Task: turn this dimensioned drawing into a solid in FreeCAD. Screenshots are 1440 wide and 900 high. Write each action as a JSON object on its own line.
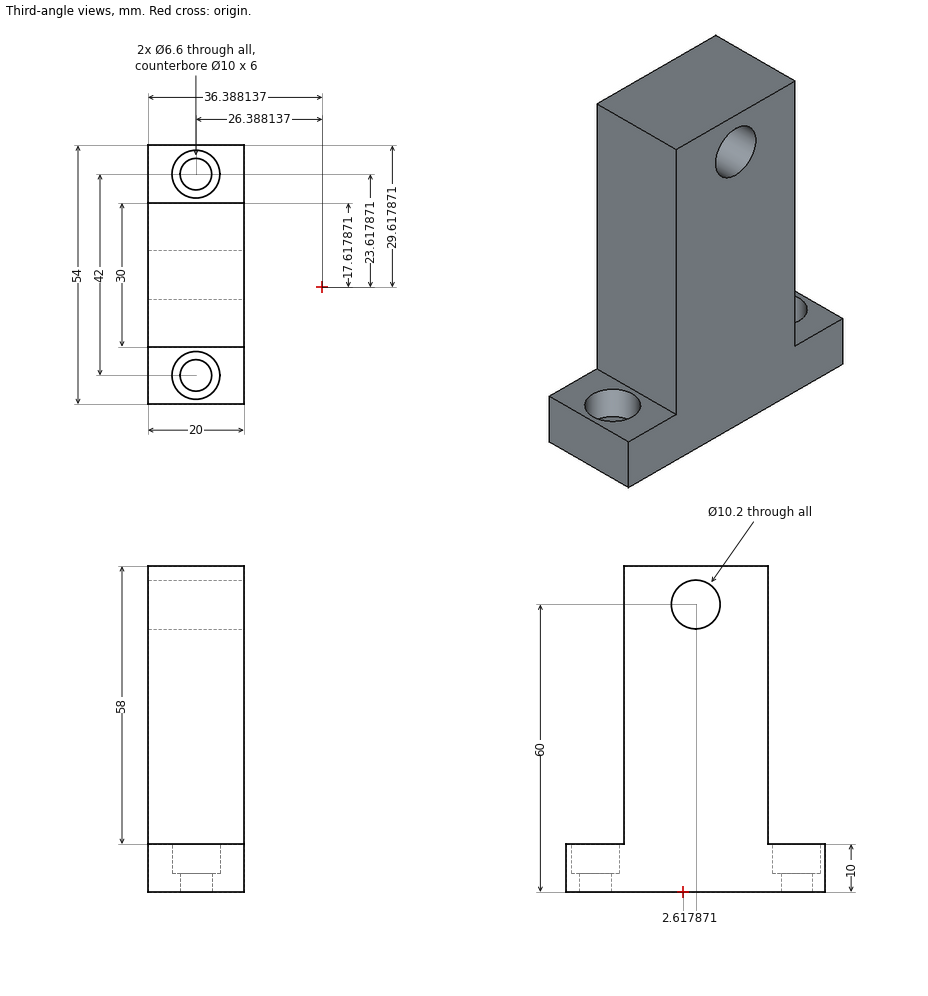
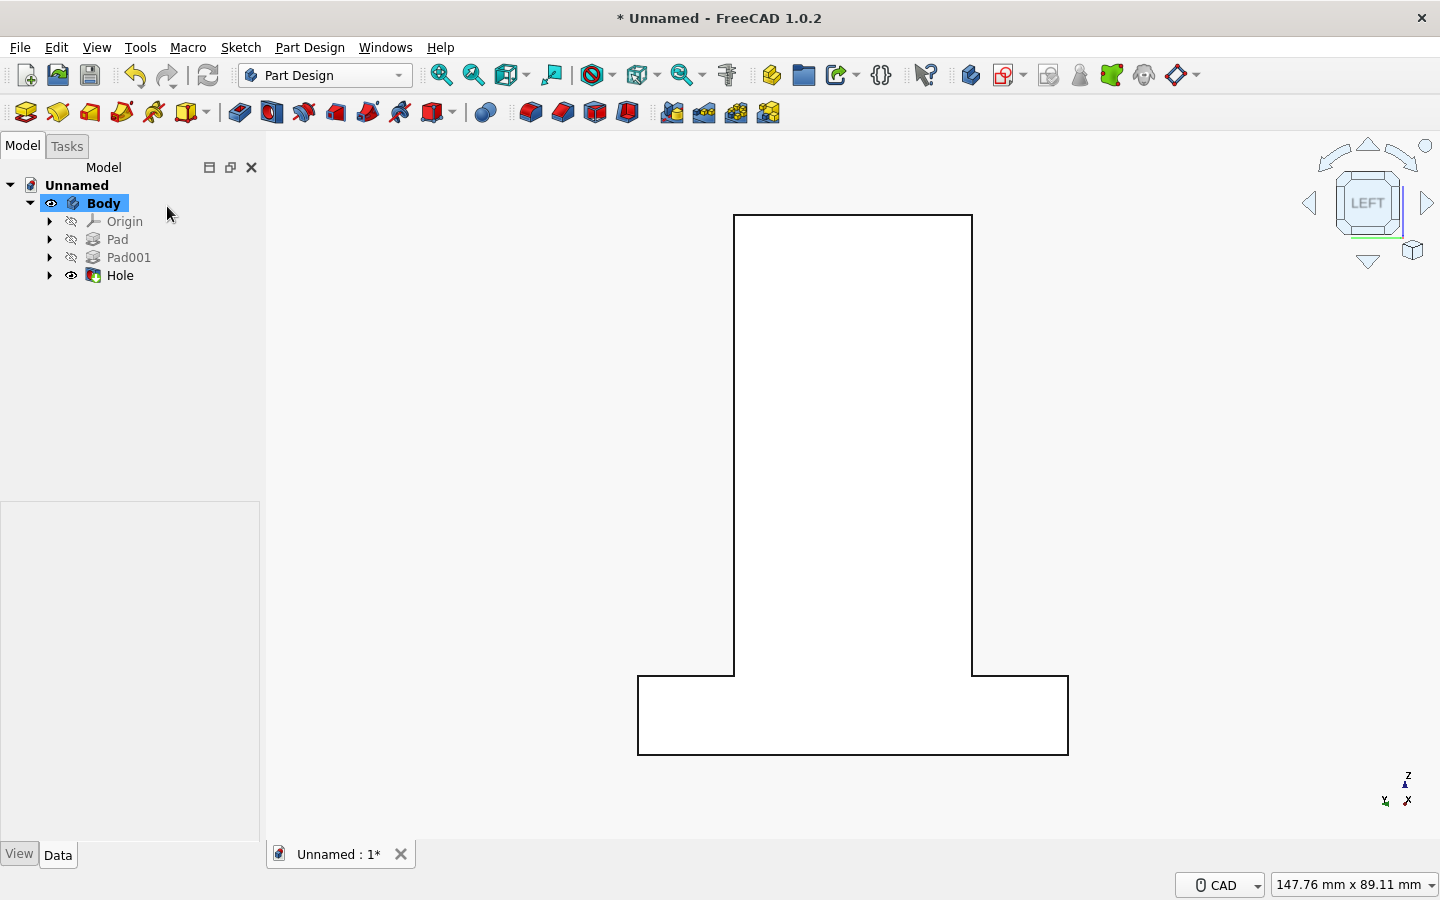
{"action": "left_click", "coordinate": [853, 407]}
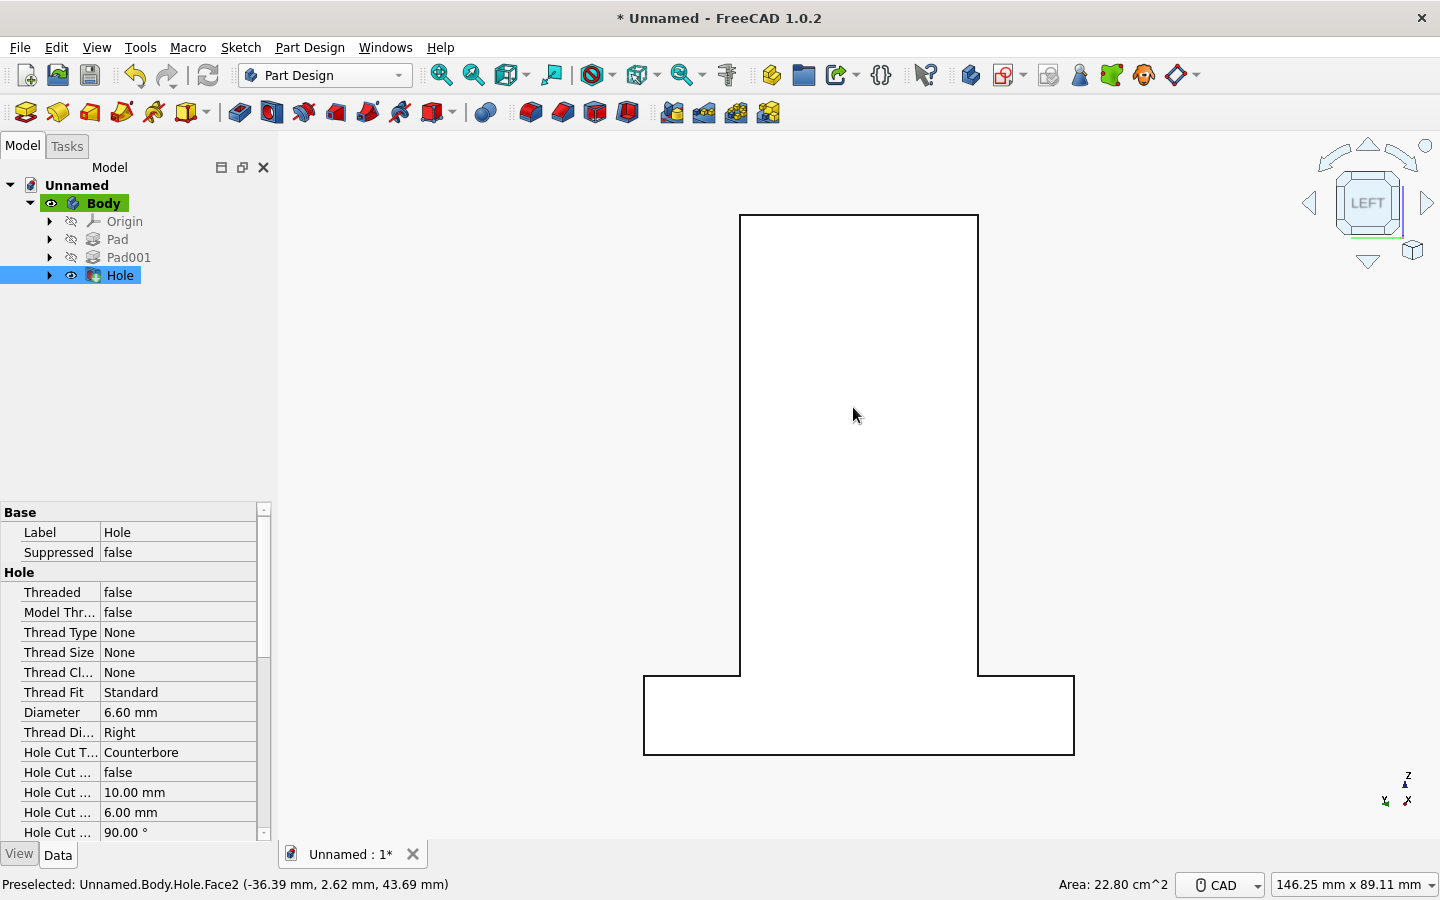
{"action": "left_click", "coordinate": [1004, 76]}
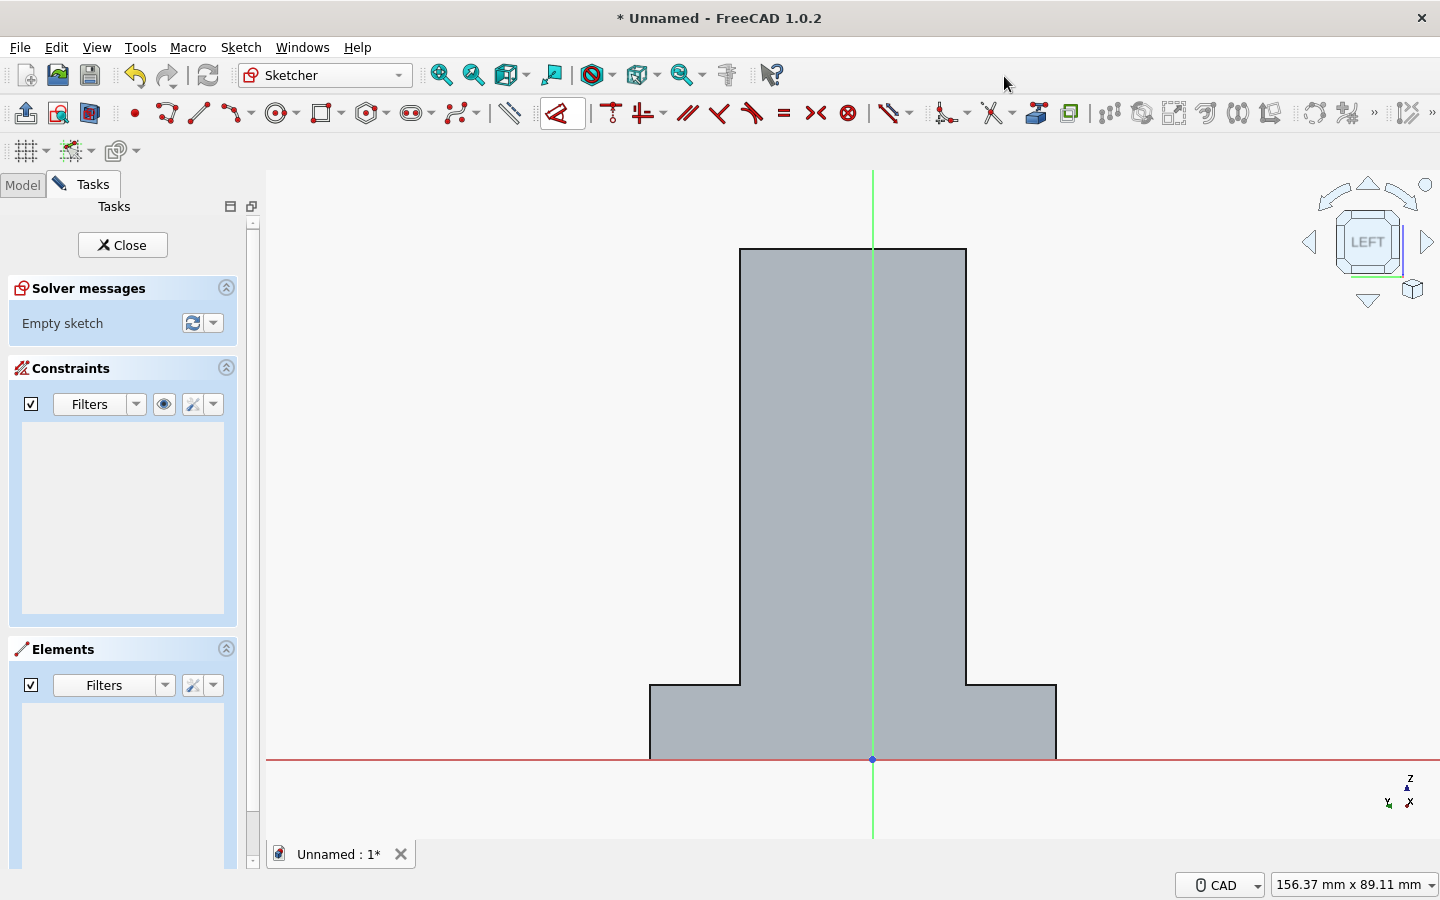
{"action": "scroll", "coordinate": [867, 271], "scroll_direction": "up", "scroll_amount": 9}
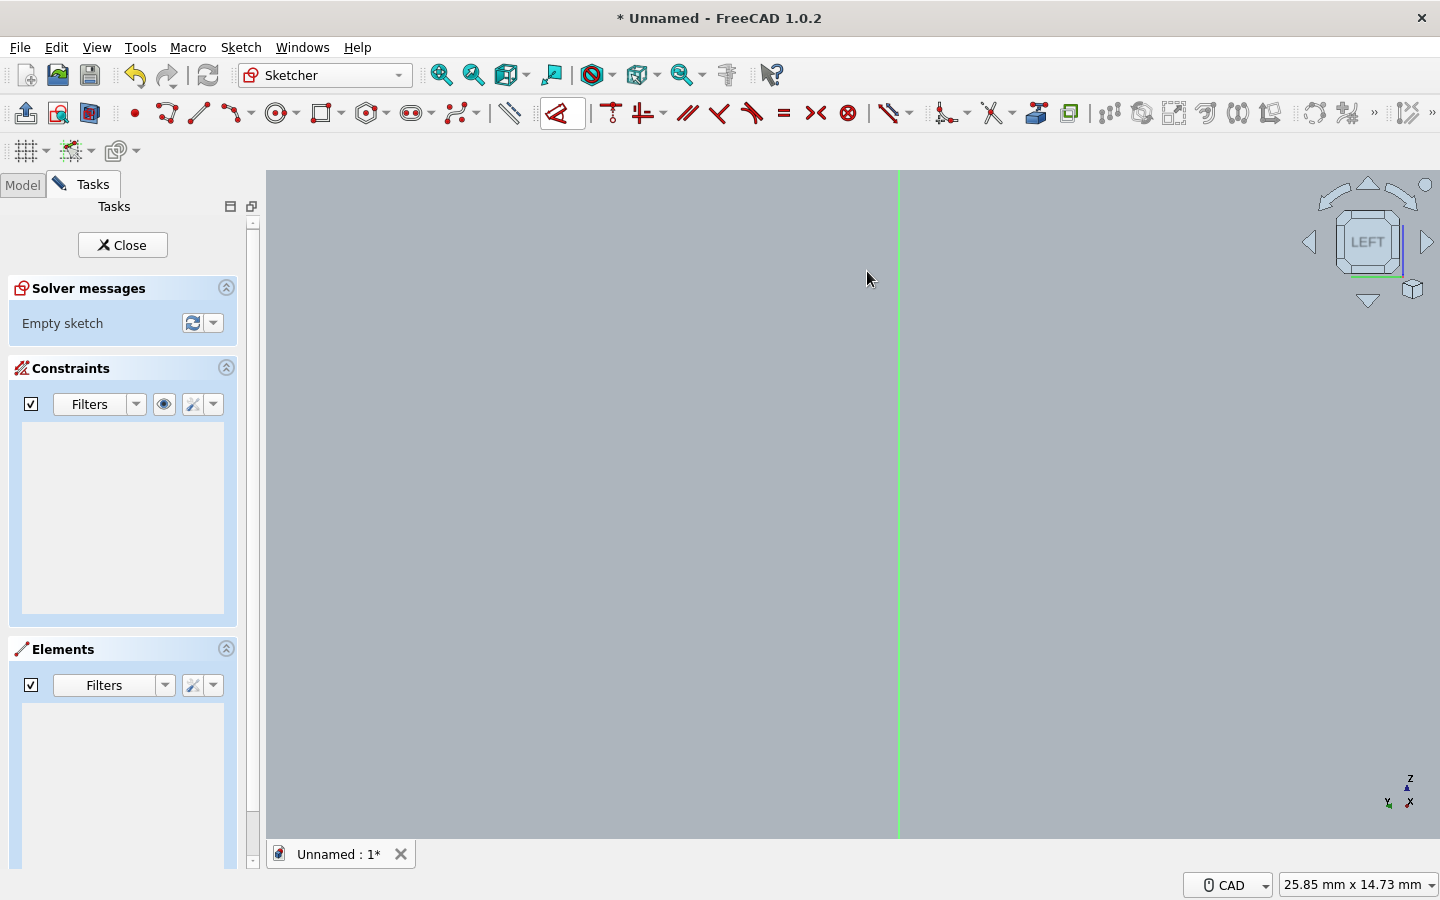
{"action": "left_click", "coordinate": [276, 114]}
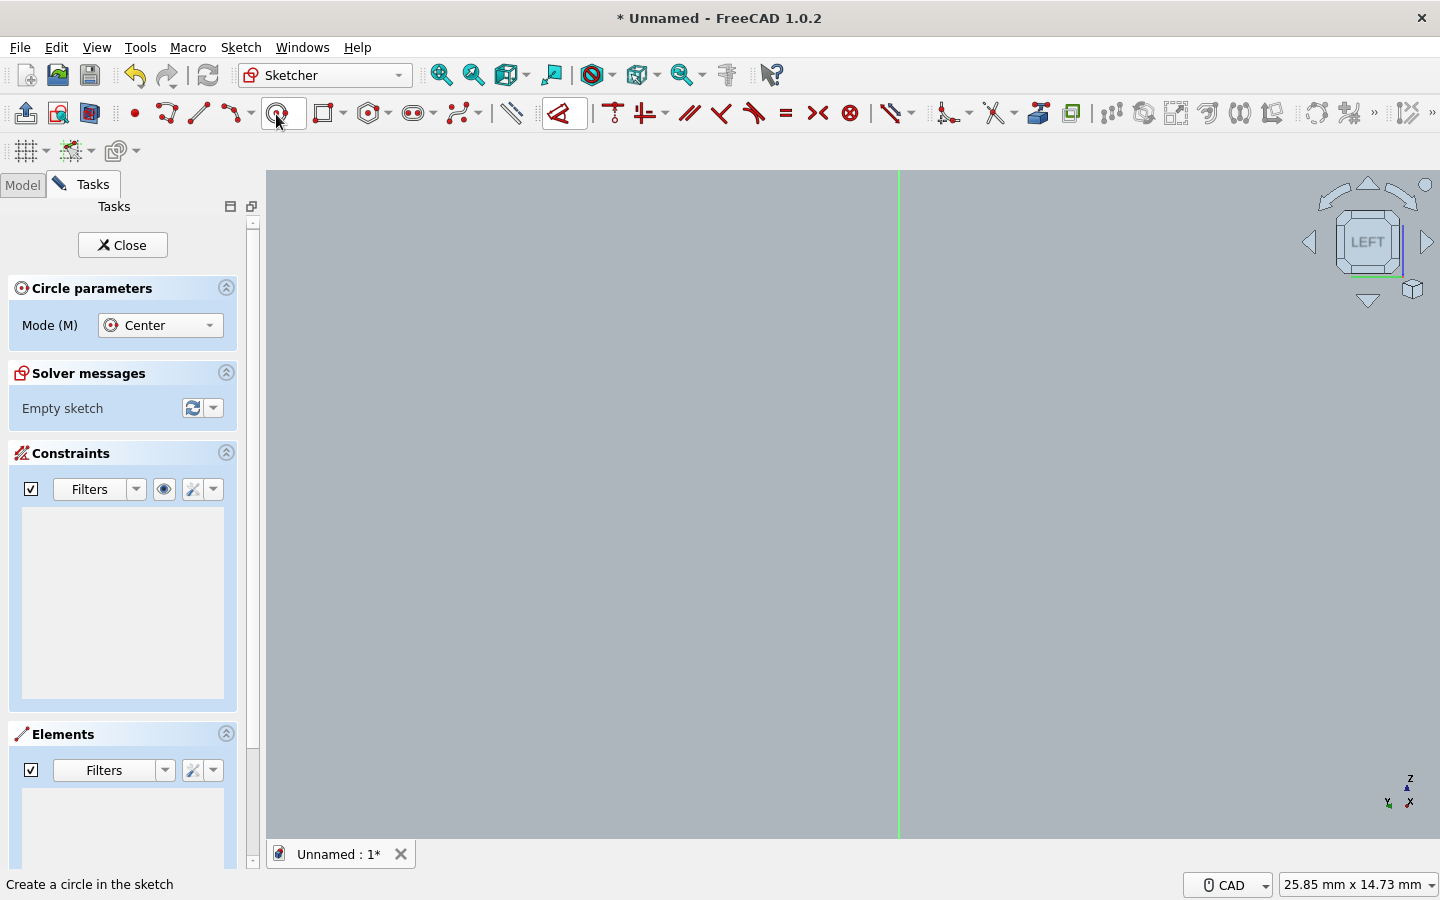
{"action": "left_click", "coordinate": [780, 502]}
{"action": "left_click", "coordinate": [944, 338]}
{"action": "key", "text": "Escape"}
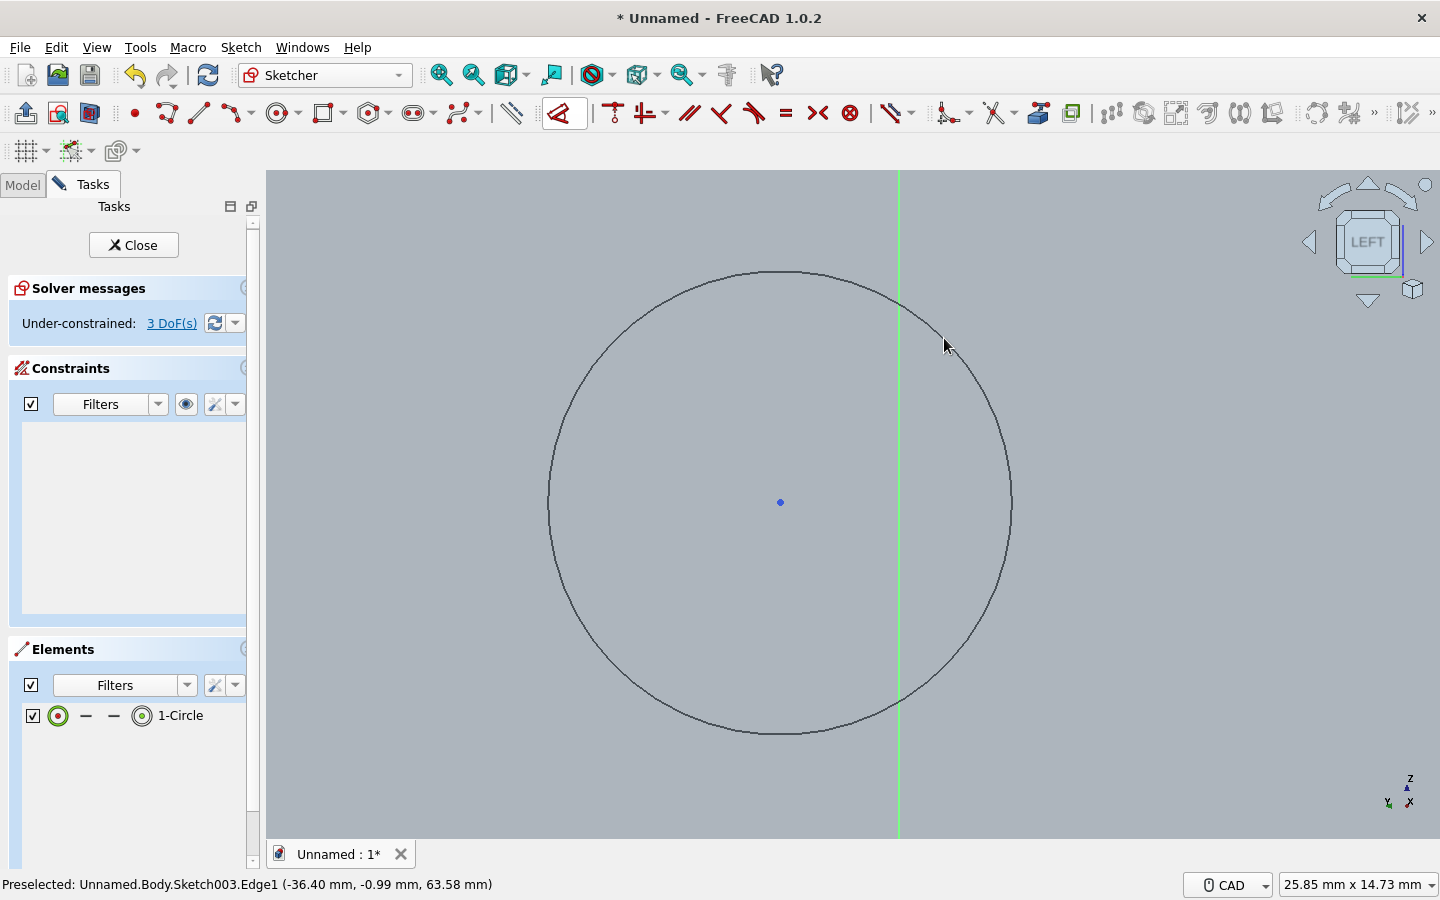
{"action": "left_click", "coordinate": [943, 338]}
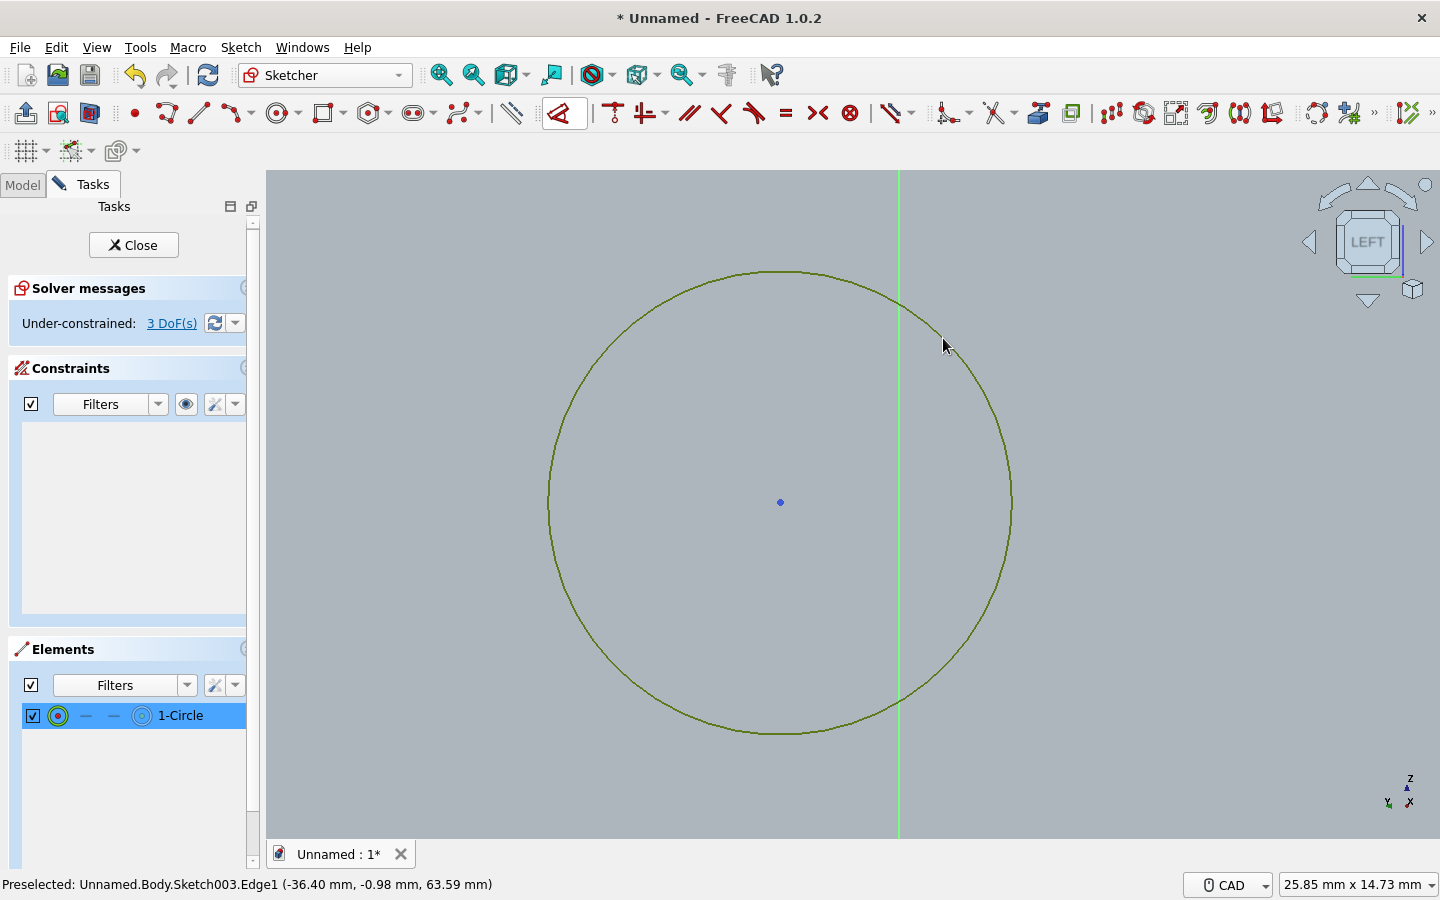
{"action": "left_click", "coordinate": [582, 114]}